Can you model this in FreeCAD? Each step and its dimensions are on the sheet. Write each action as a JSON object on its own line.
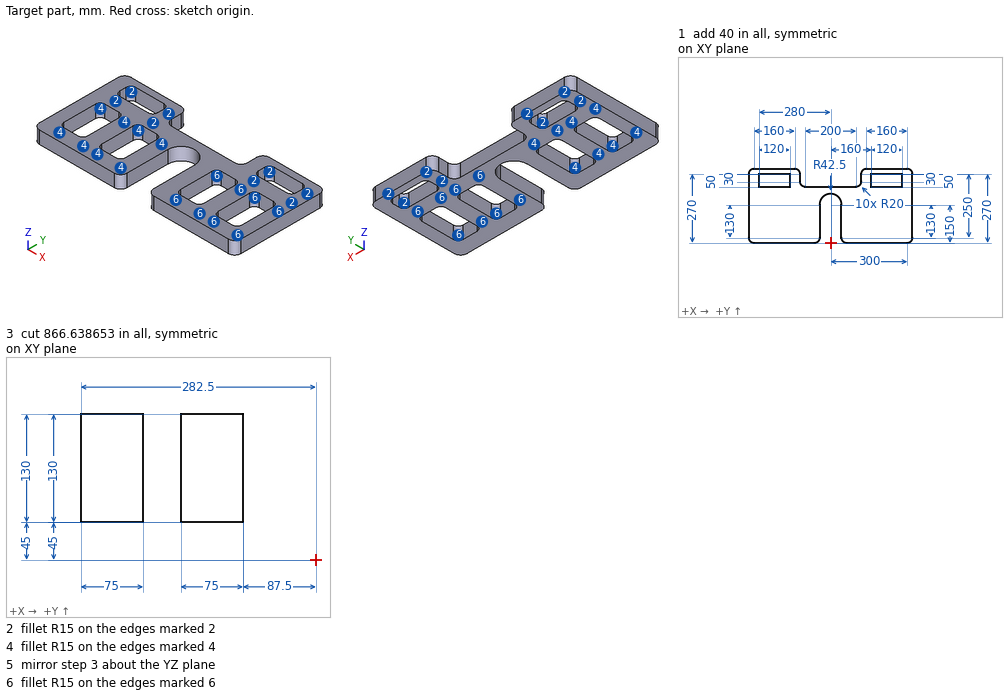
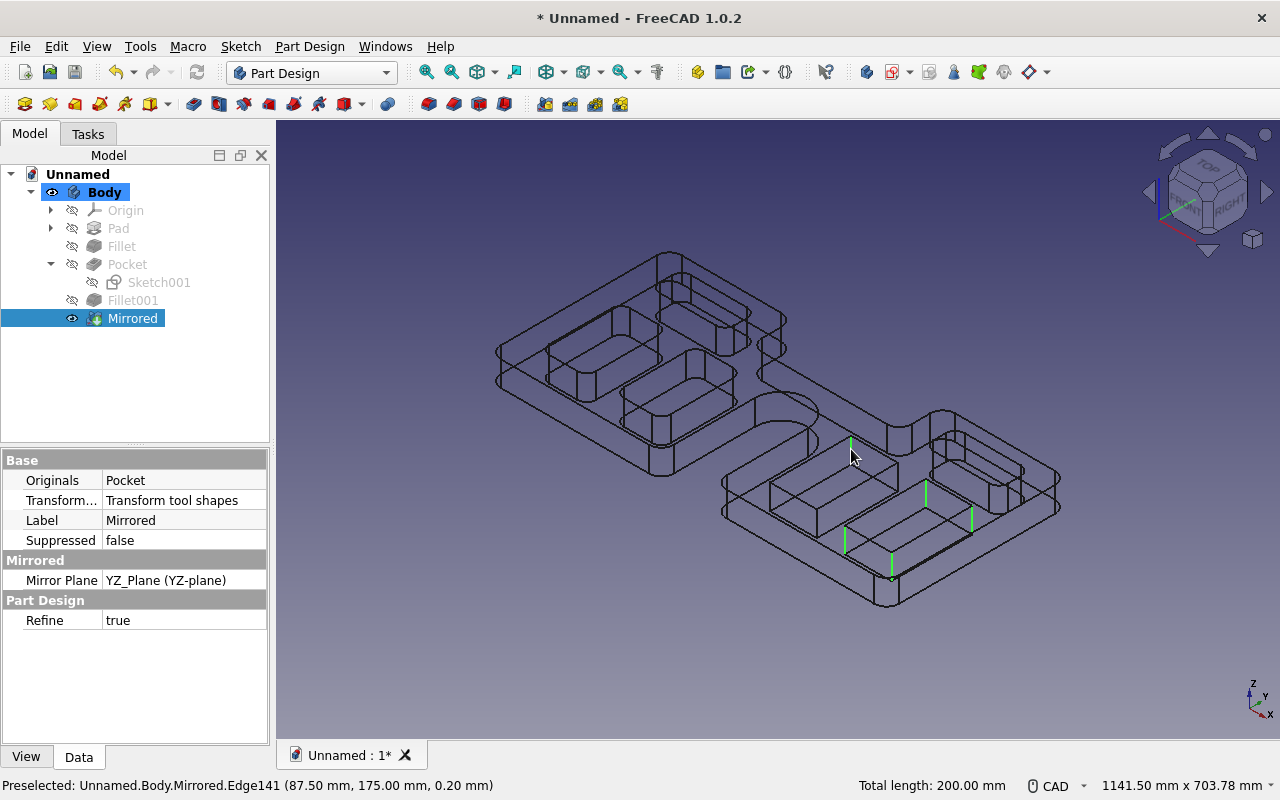
{"action": "left_click", "coordinate": [770, 496], "text": "ctrl"}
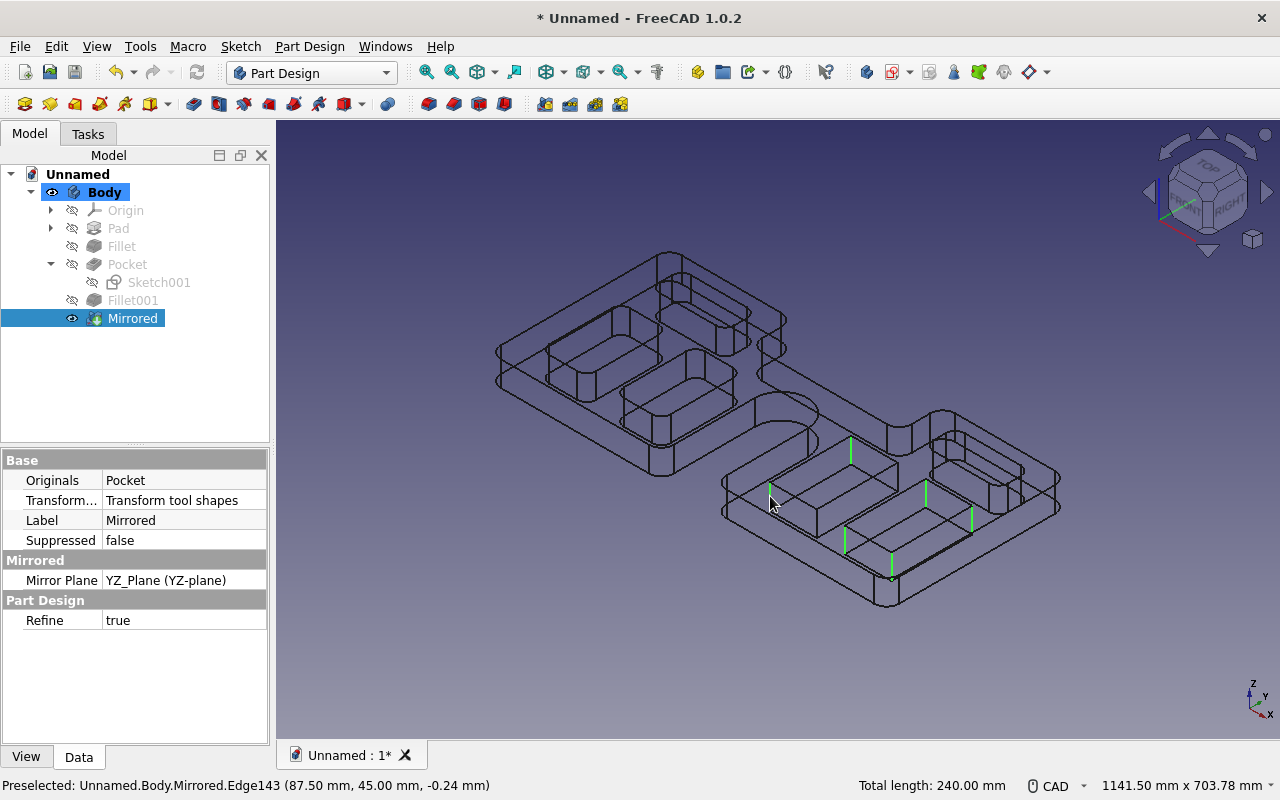
{"action": "left_click", "coordinate": [817, 523], "text": "ctrl"}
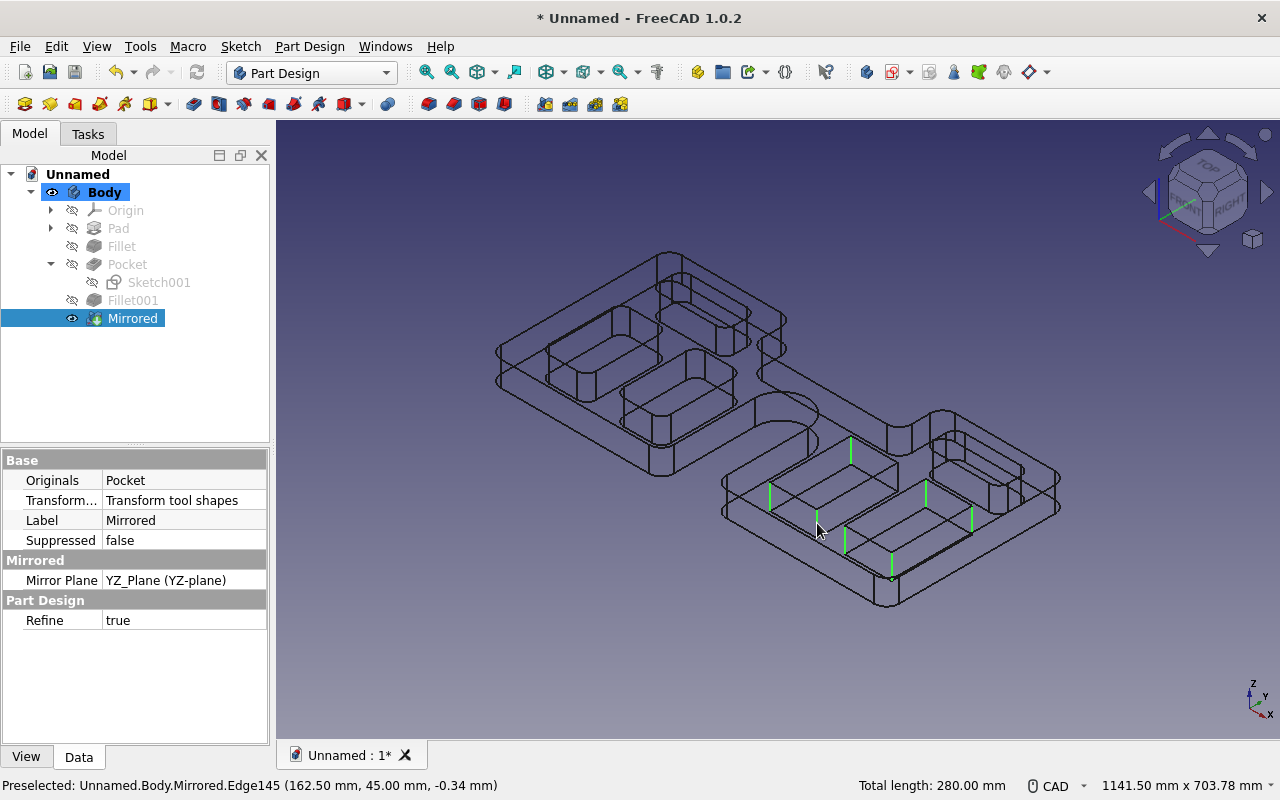
{"action": "left_click", "coordinate": [898, 476], "text": "ctrl"}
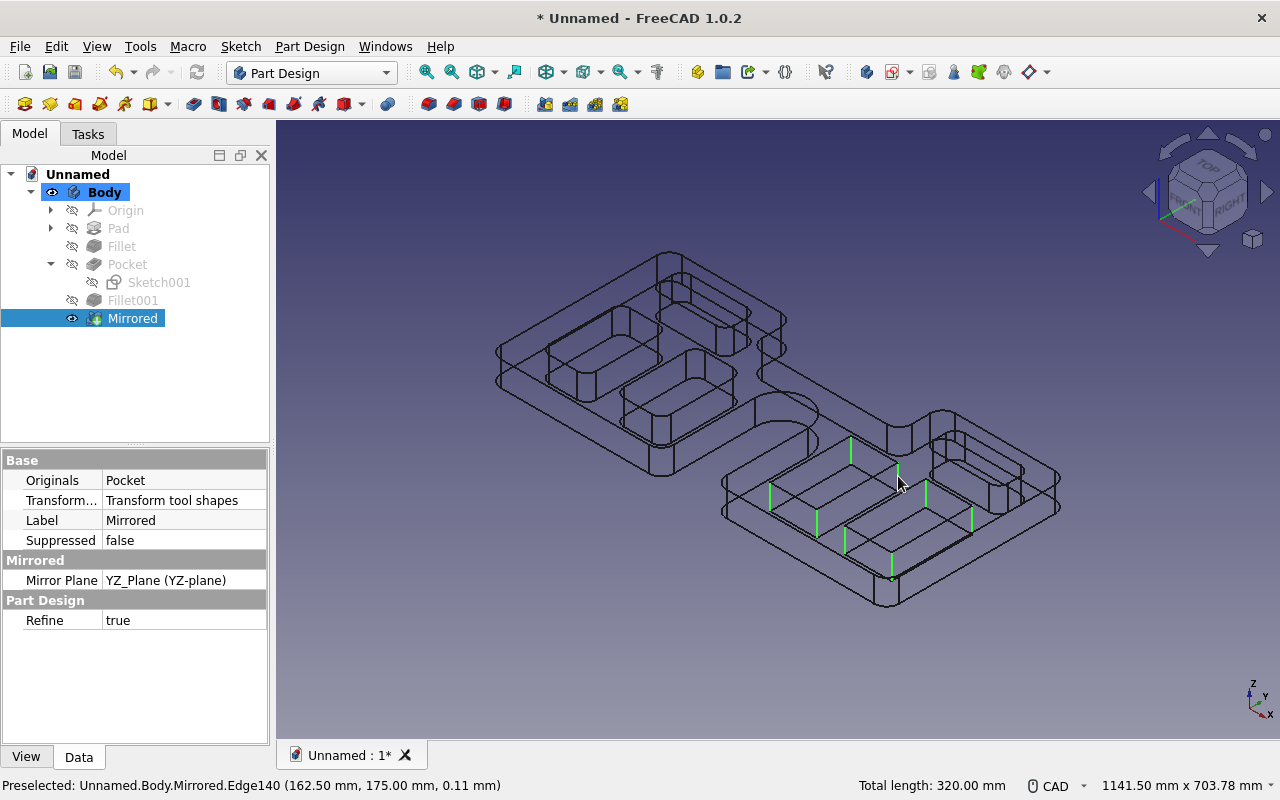
{"action": "key", "text": "v 1"}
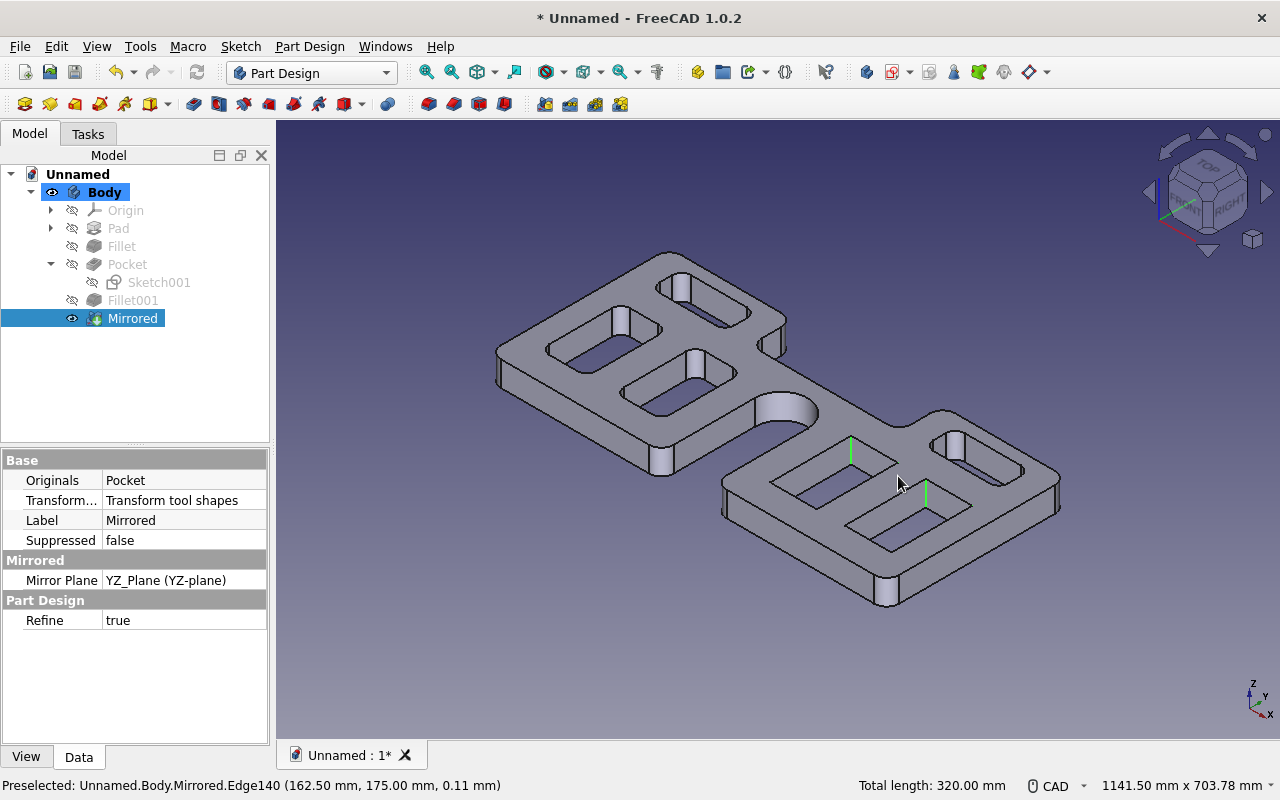
{"action": "left_click", "coordinate": [429, 104]}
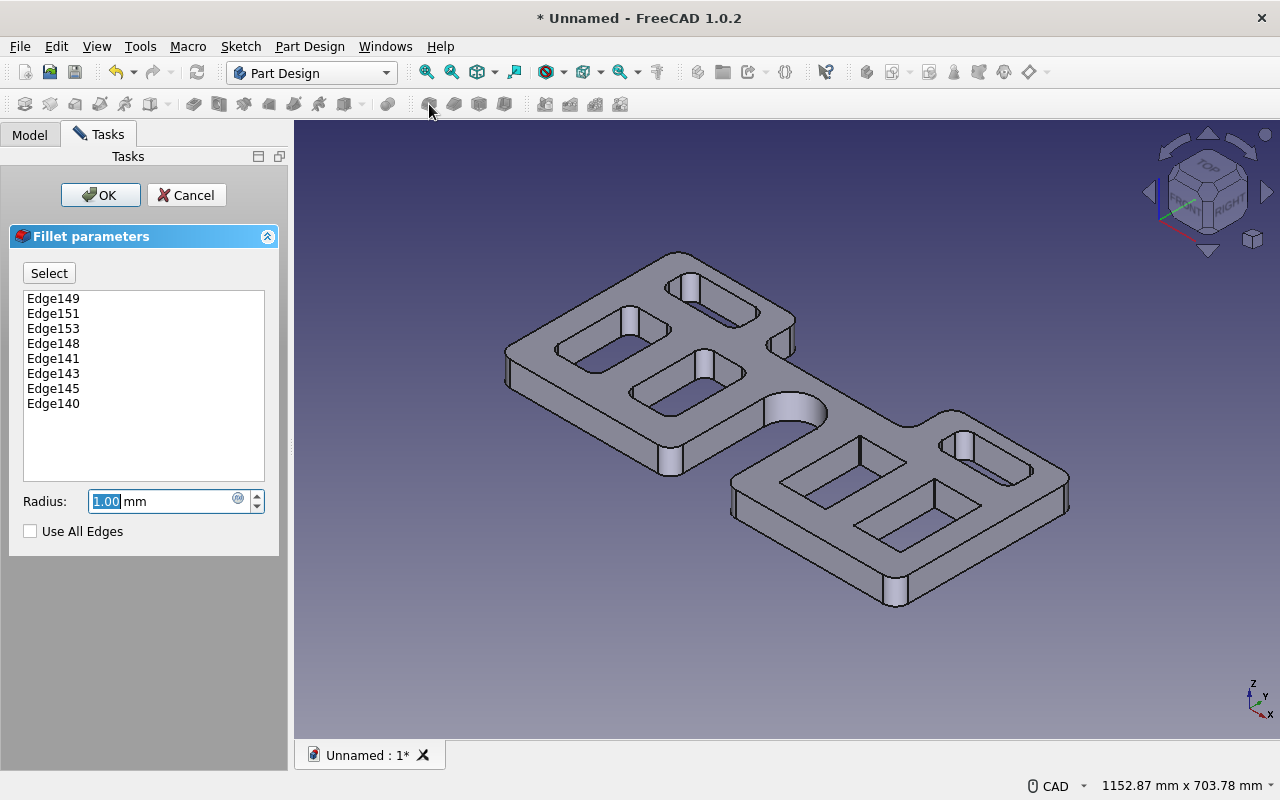
{"action": "type", "text": "15"}
{"action": "key", "text": "Tab"}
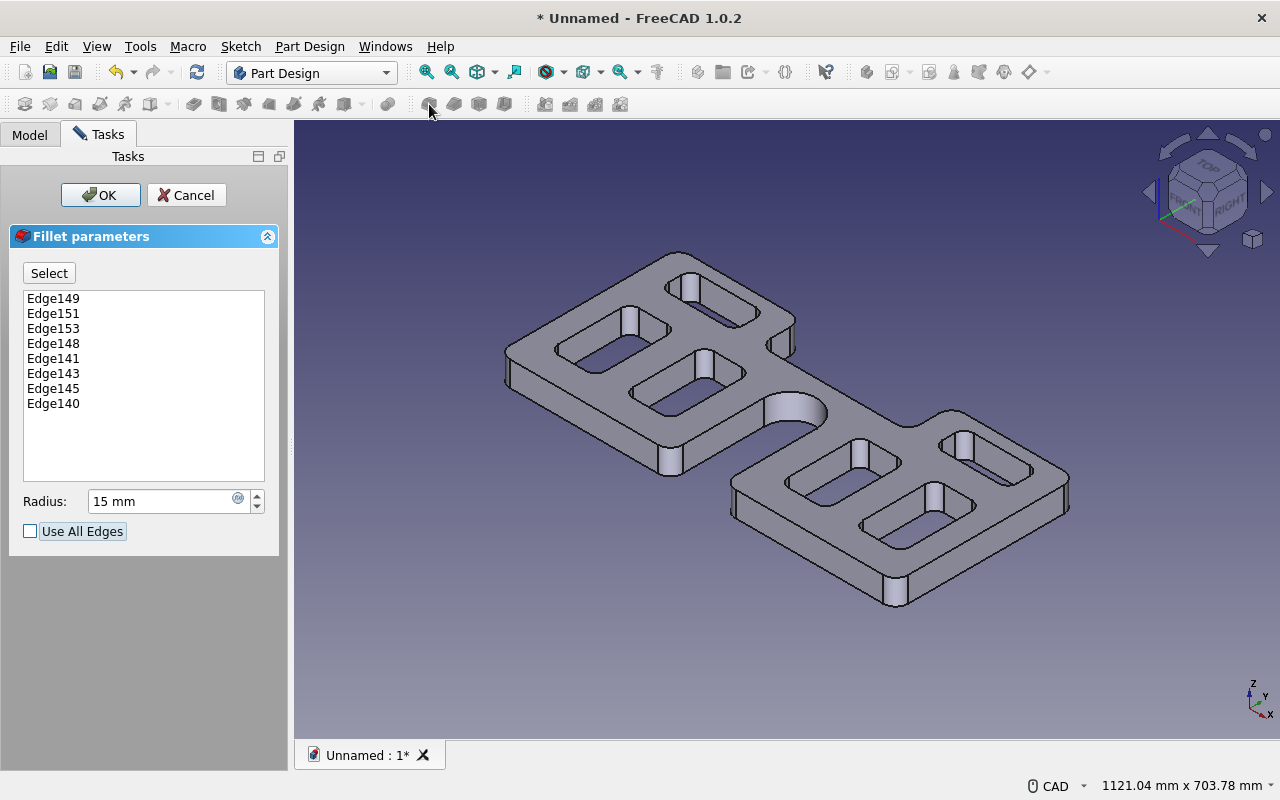
{"action": "left_click", "coordinate": [101, 195]}